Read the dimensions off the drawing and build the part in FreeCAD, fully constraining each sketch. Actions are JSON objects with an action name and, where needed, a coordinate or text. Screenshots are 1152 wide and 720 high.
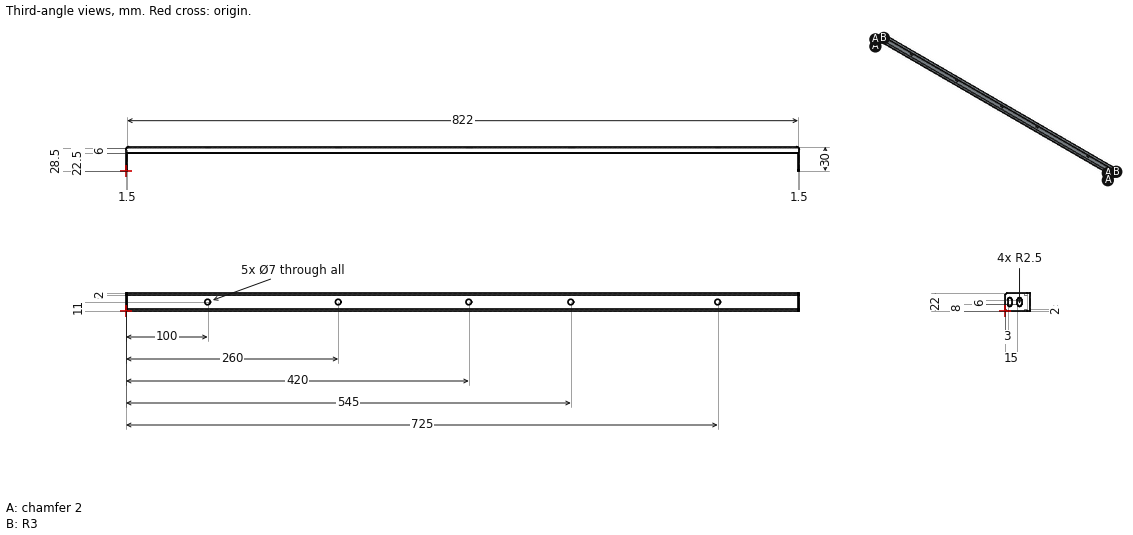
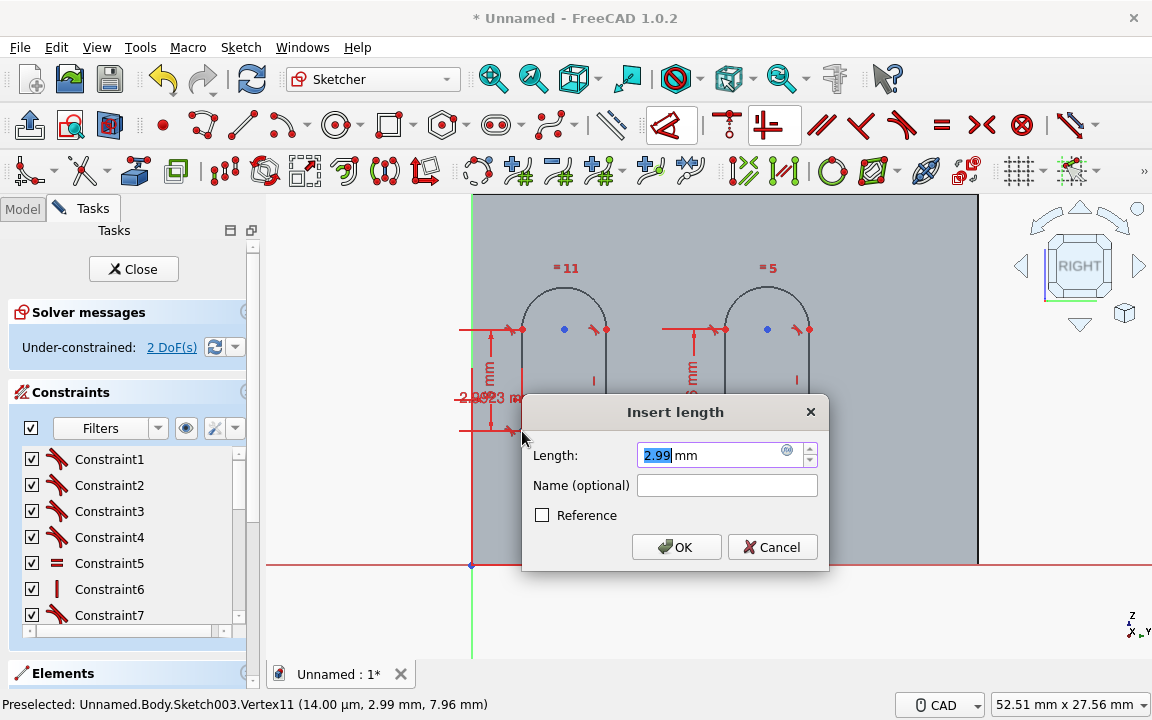
{"action": "type", "text": "3"}
{"action": "key", "text": "Return"}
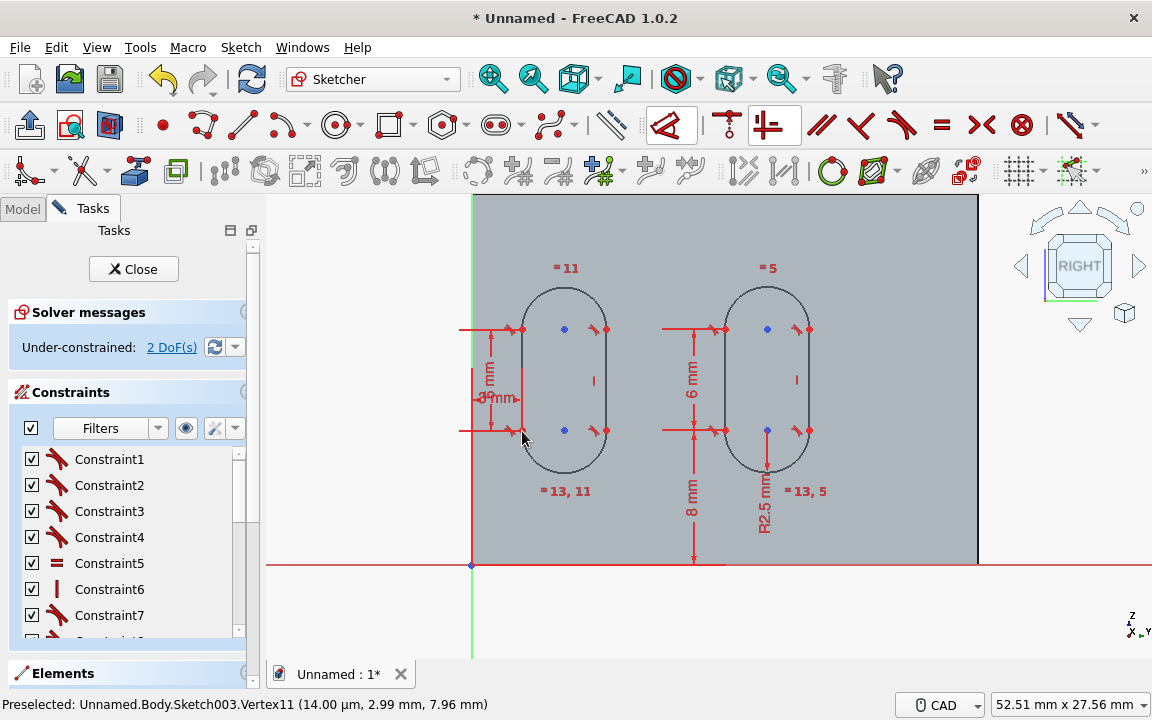
{"action": "left_click", "coordinate": [522, 431]}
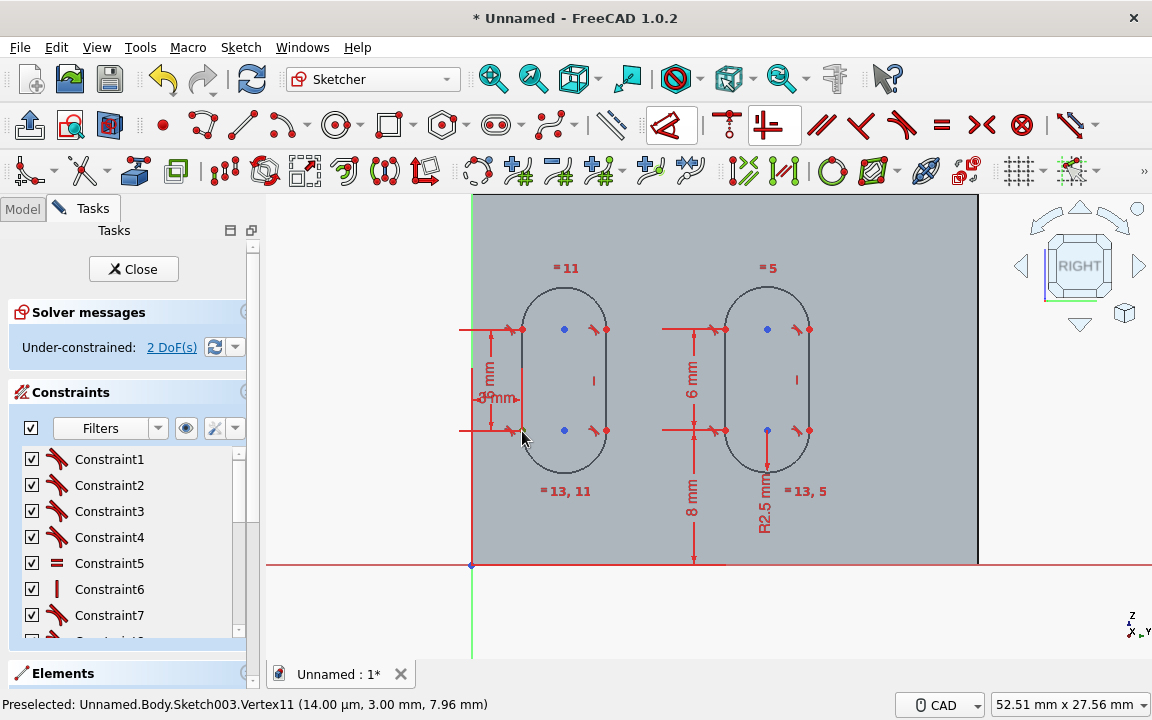
{"action": "key", "text": "i"}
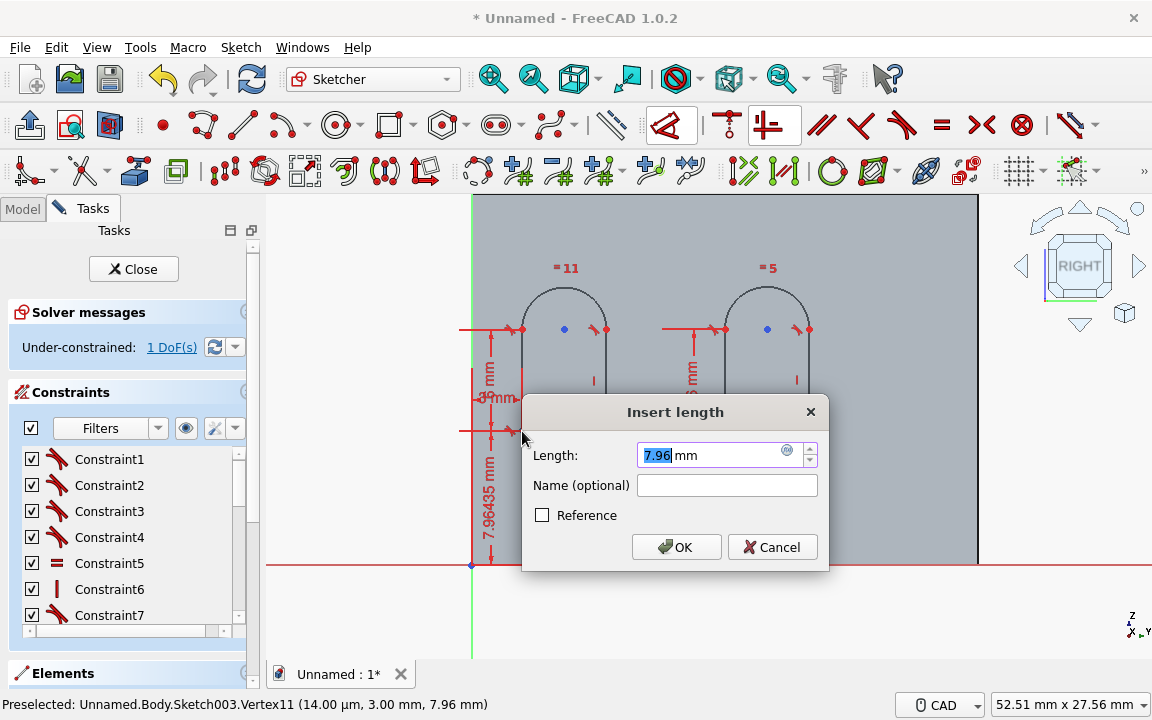
{"action": "type", "text": "8"}
{"action": "key", "text": "Return"}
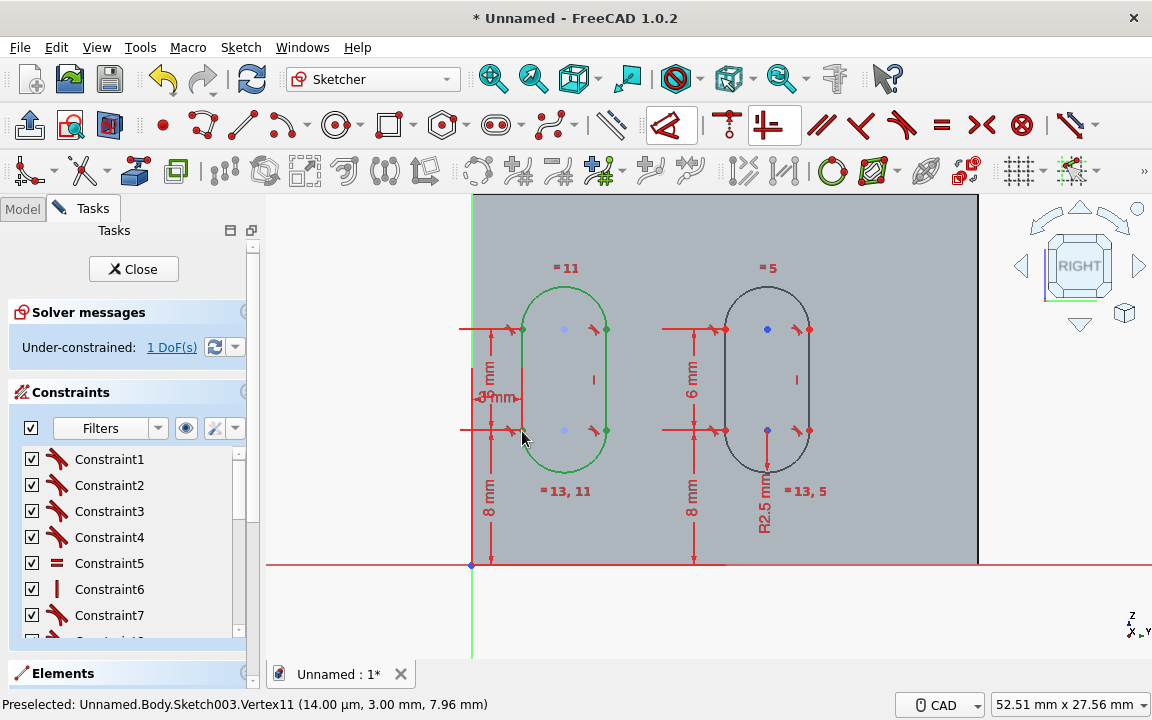
{"action": "left_click", "coordinate": [725, 430]}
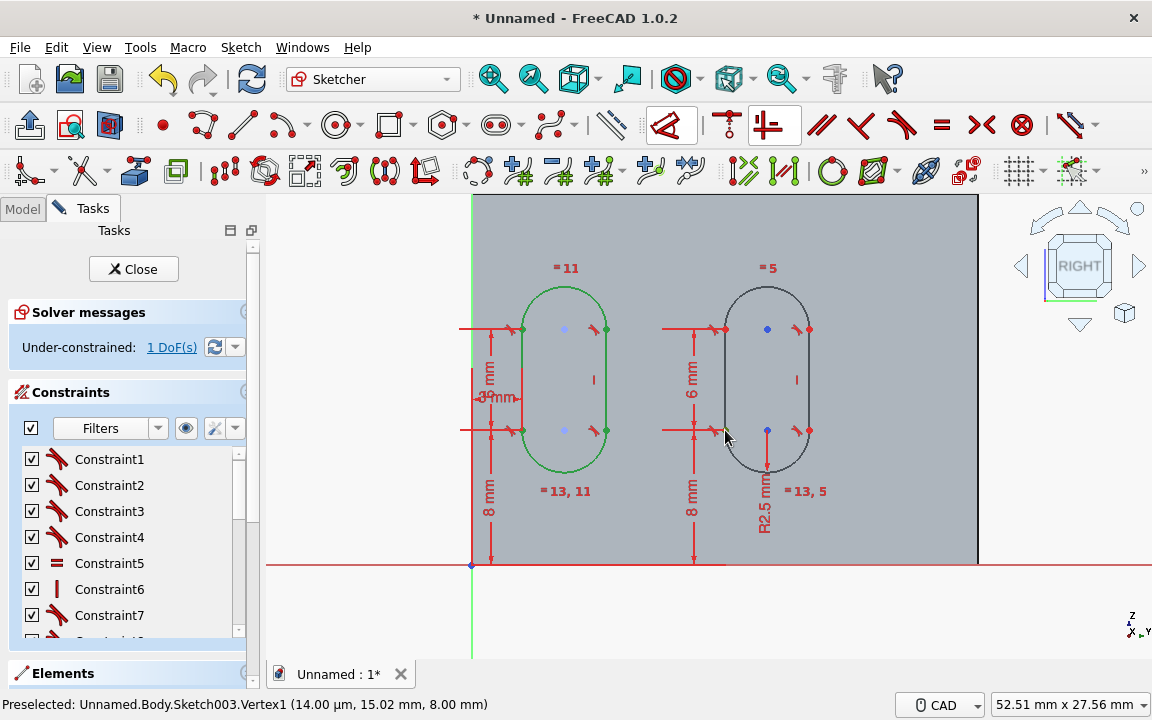
{"action": "key", "text": "l"}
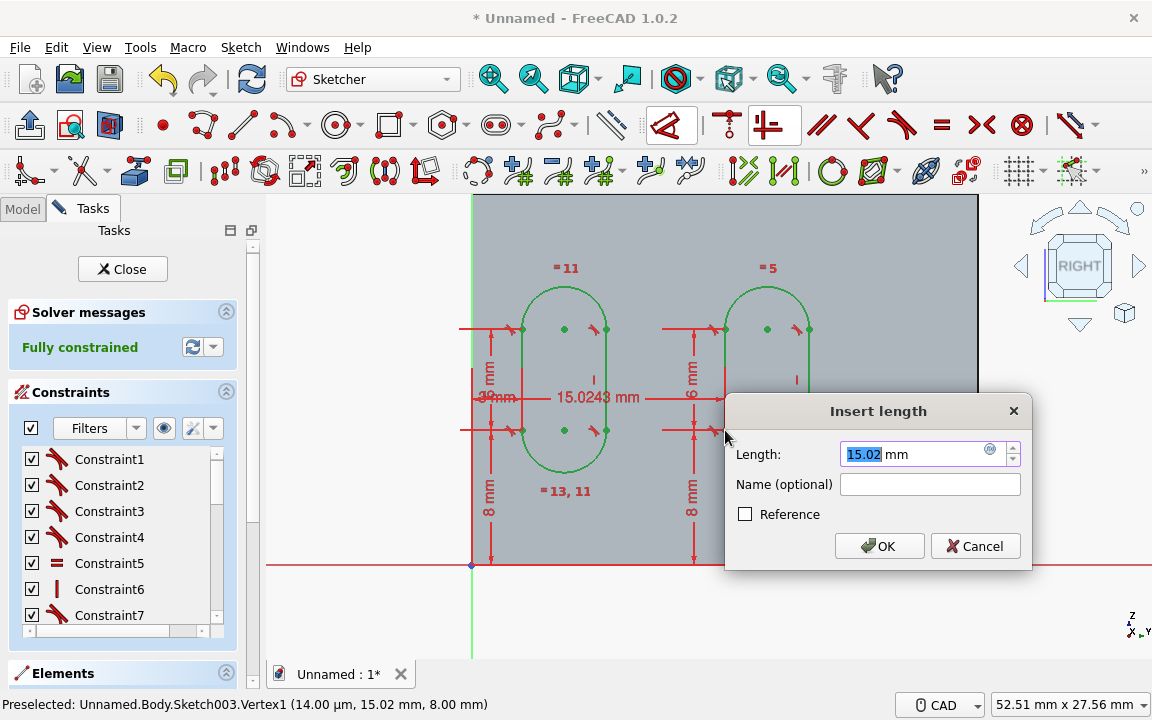
{"action": "type", "text": "15"}
{"action": "key", "text": "Return"}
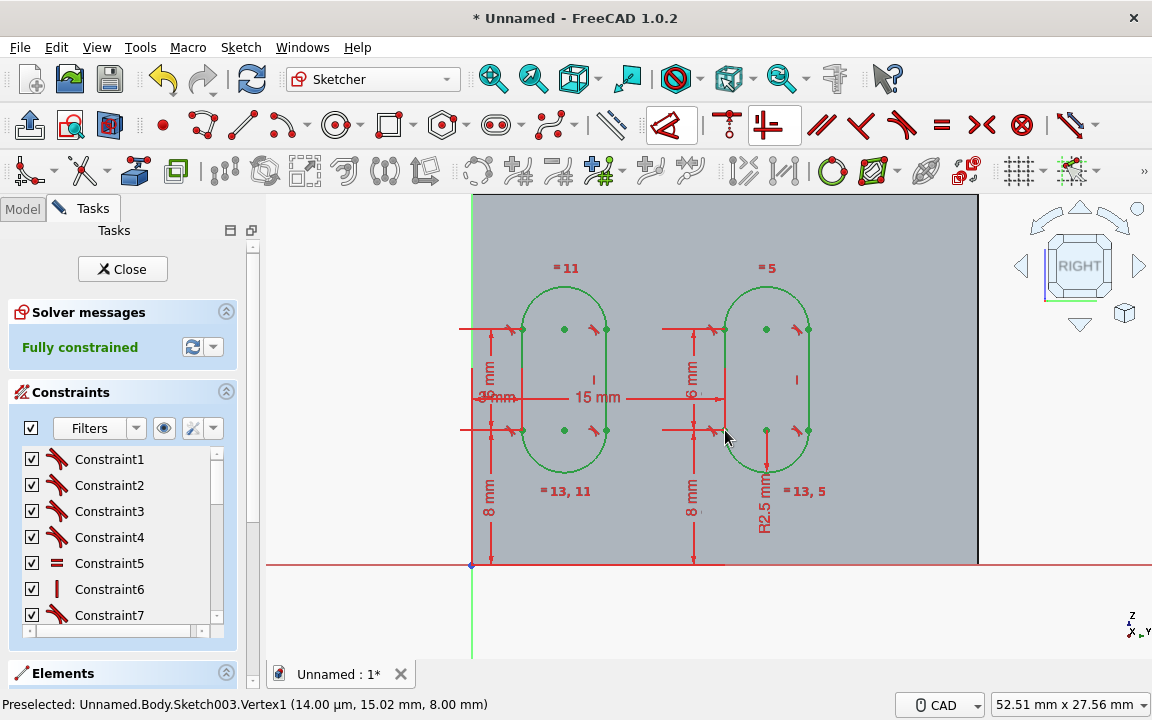
{"action": "left_click", "coordinate": [123, 269]}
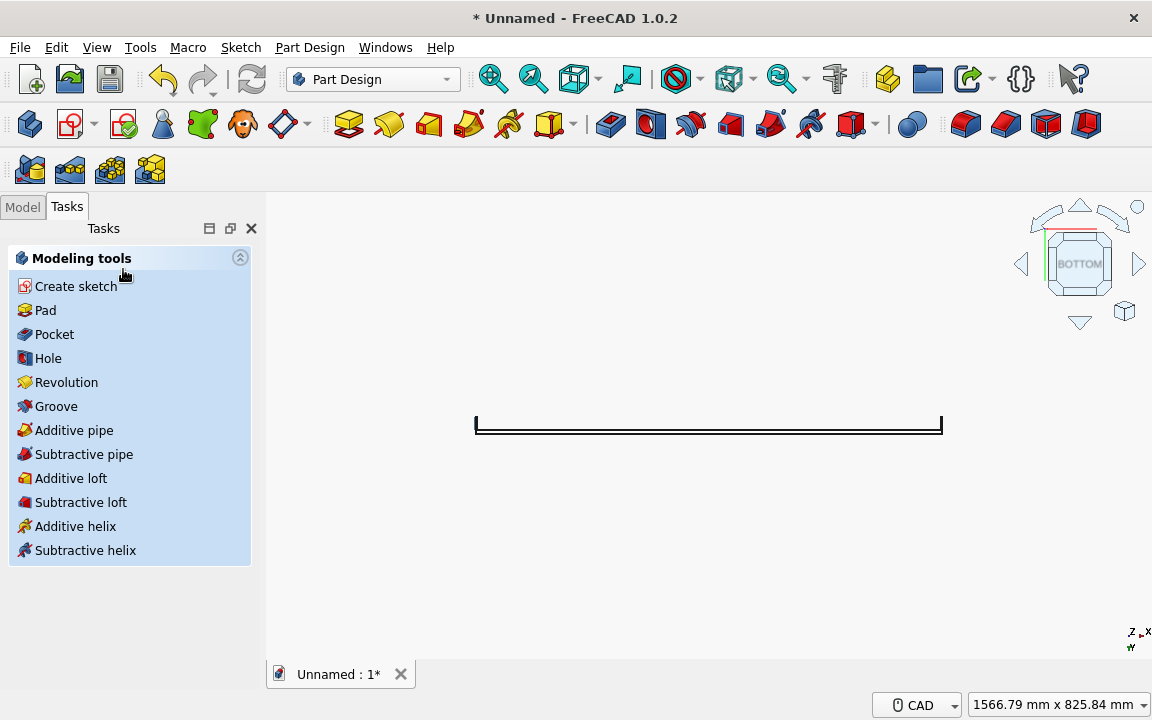
{"action": "left_click", "coordinate": [612, 124]}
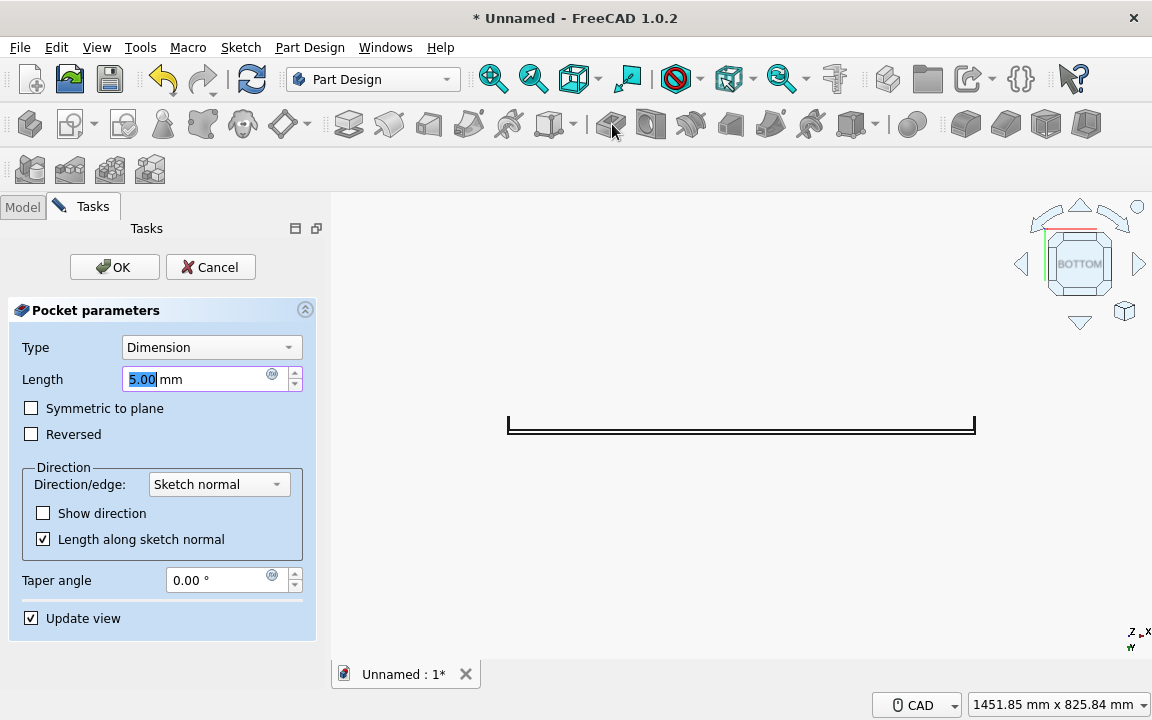
{"action": "left_click", "coordinate": [212, 348]}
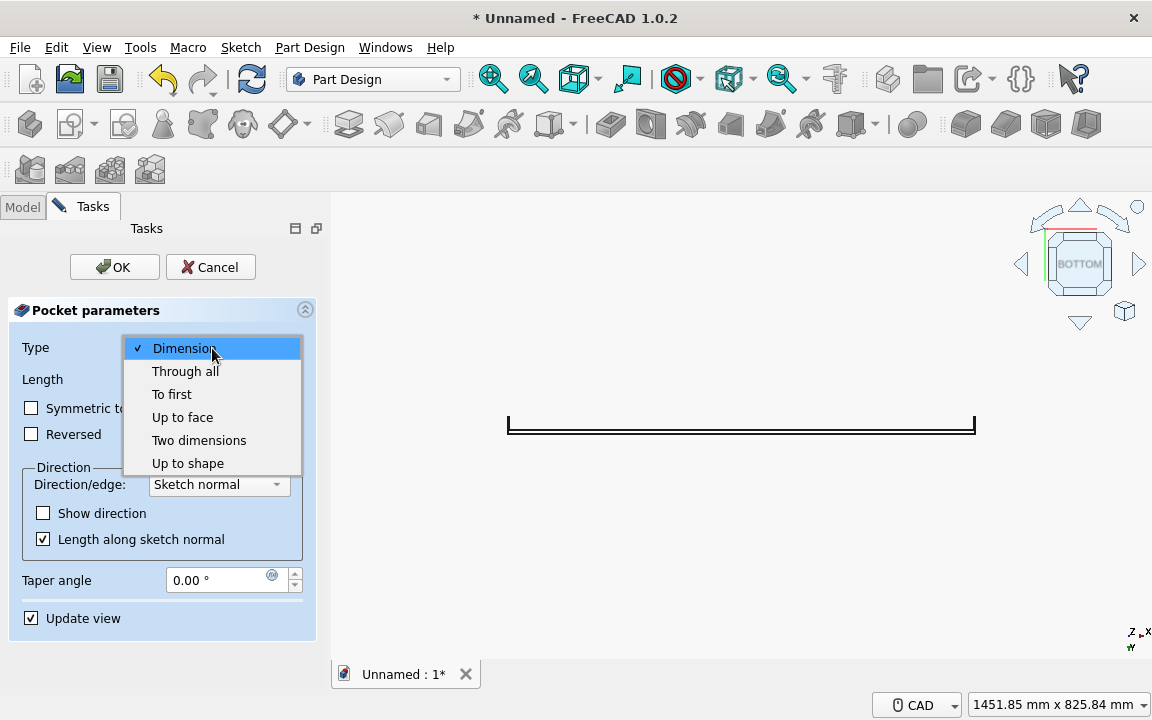
{"action": "left_click", "coordinate": [212, 372]}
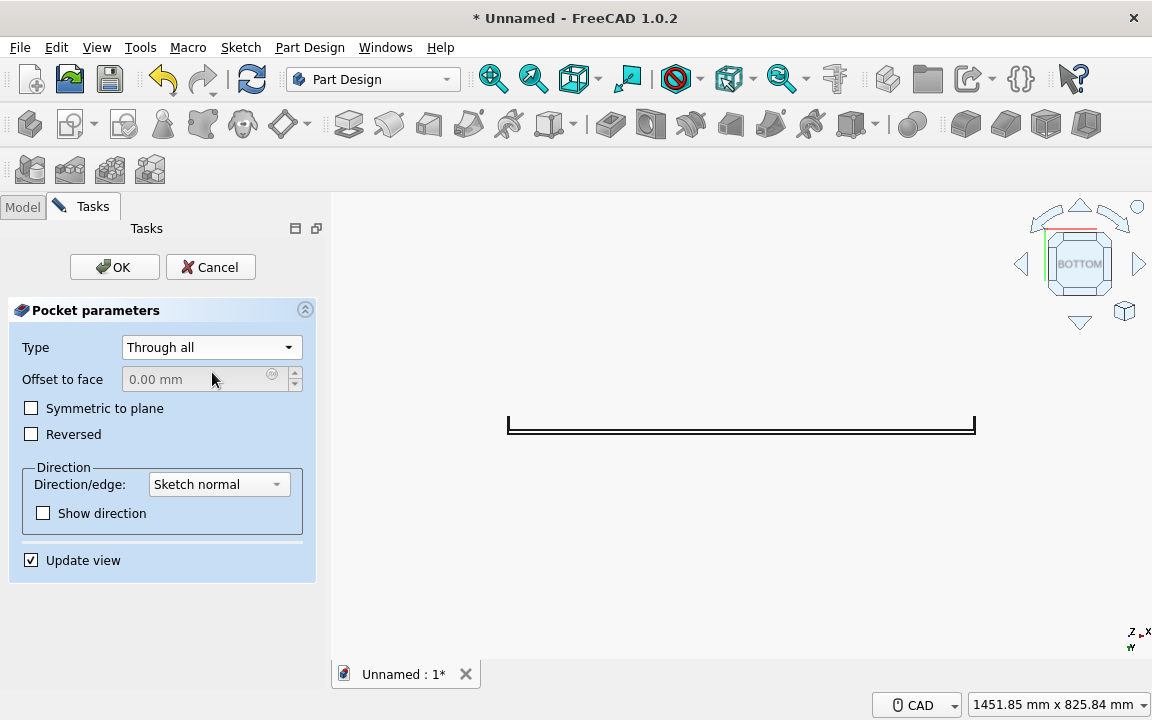
{"action": "left_click", "coordinate": [30, 434]}